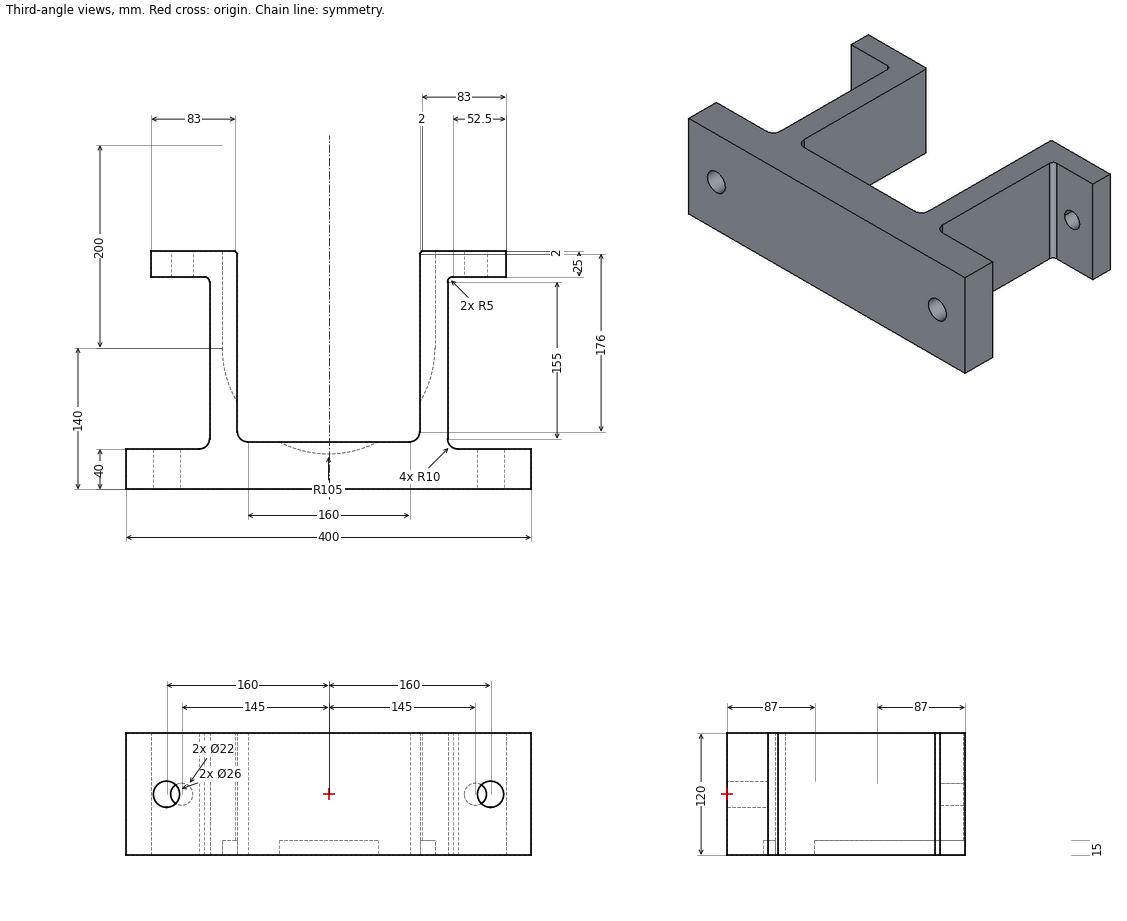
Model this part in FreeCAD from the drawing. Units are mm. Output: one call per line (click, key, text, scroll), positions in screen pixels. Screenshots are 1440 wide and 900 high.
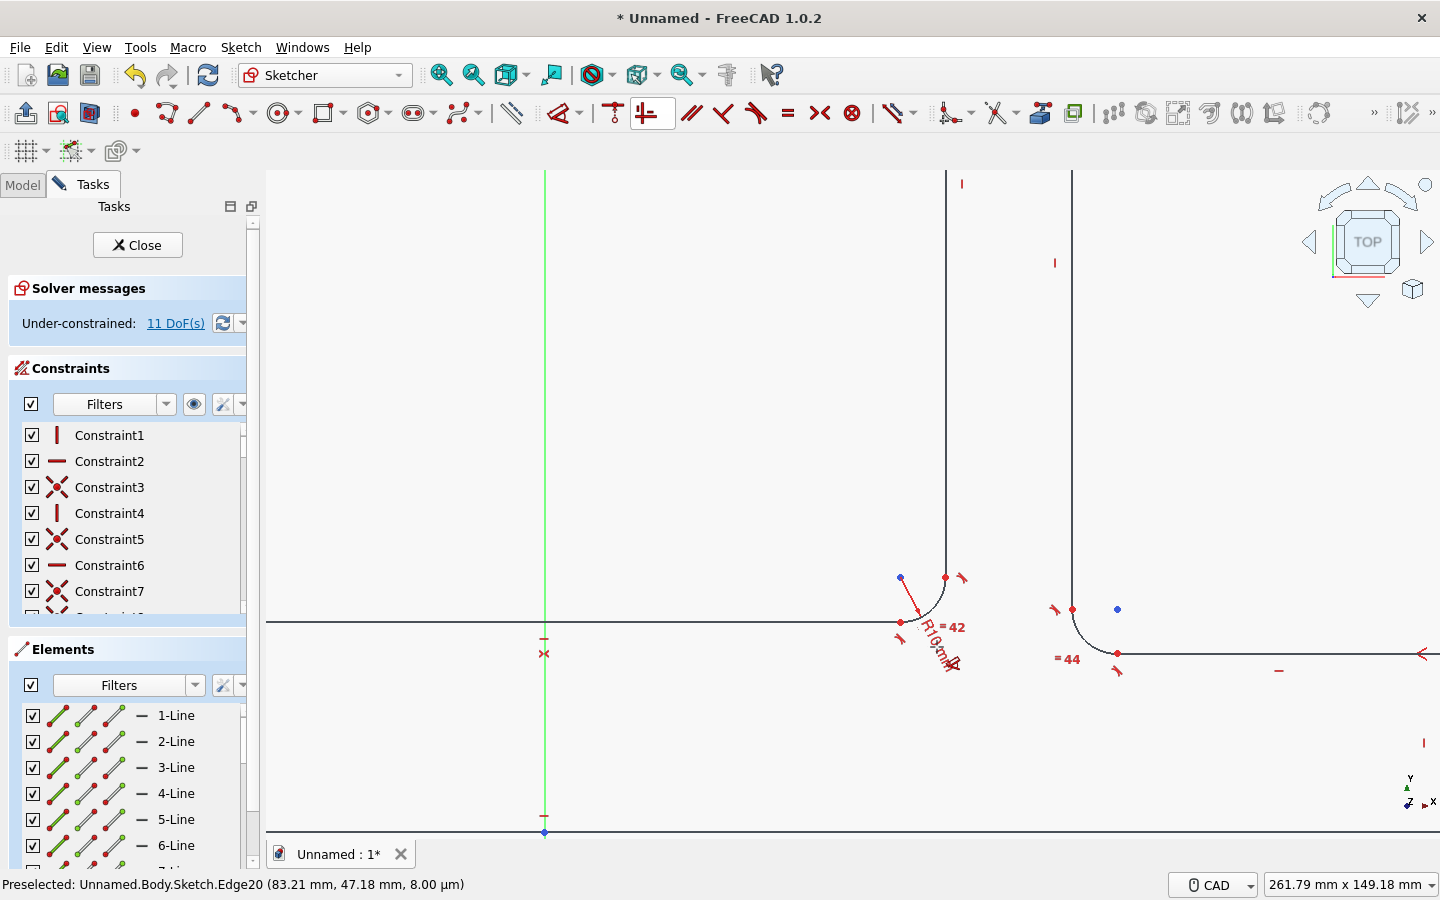
scroll(924, 621, down, 5)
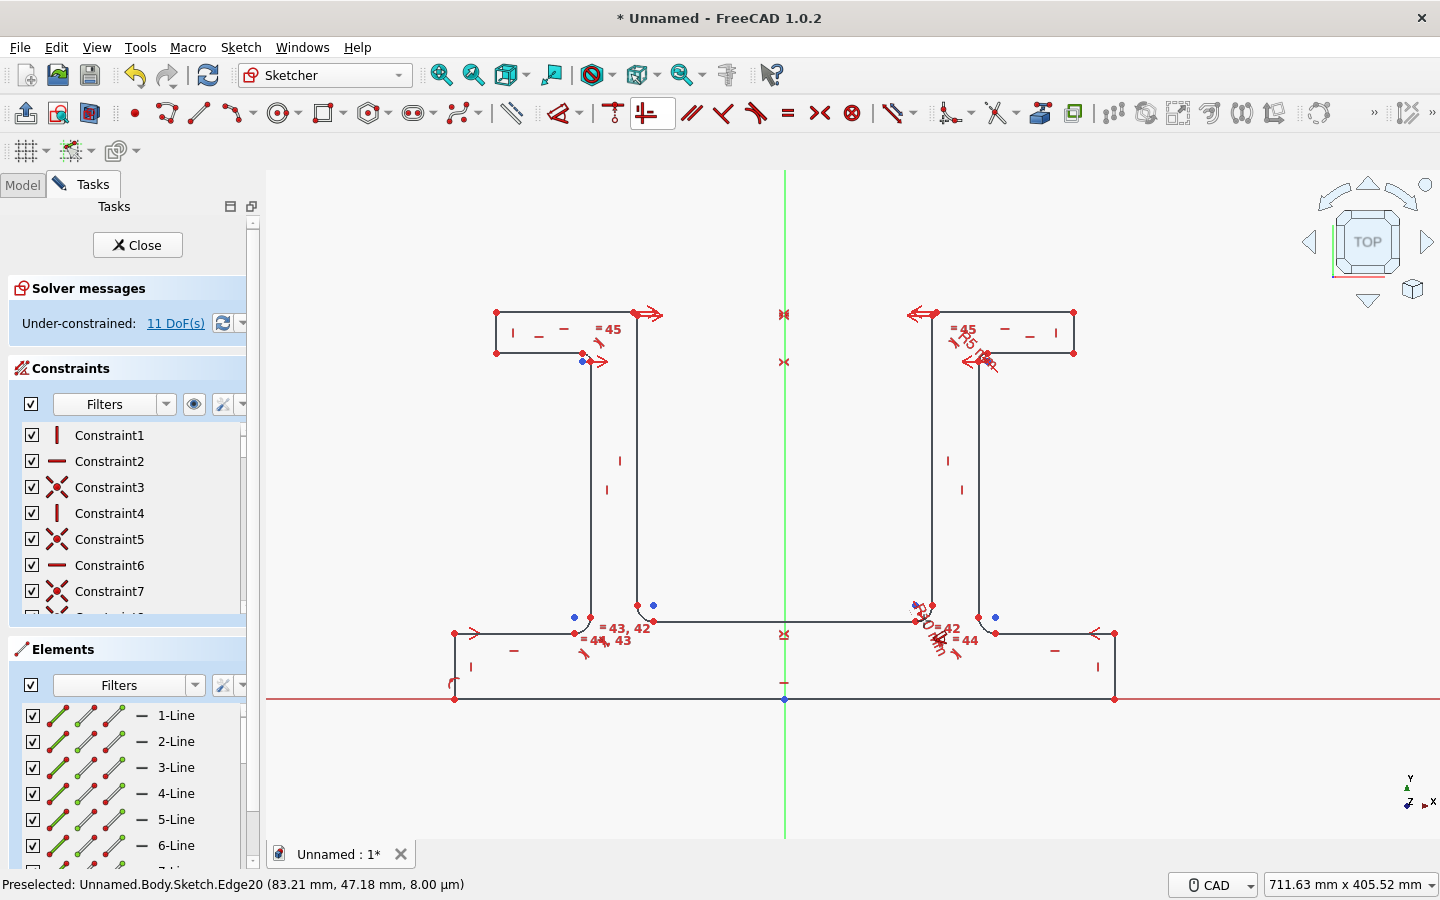
click(1074, 341)
click(1108, 333)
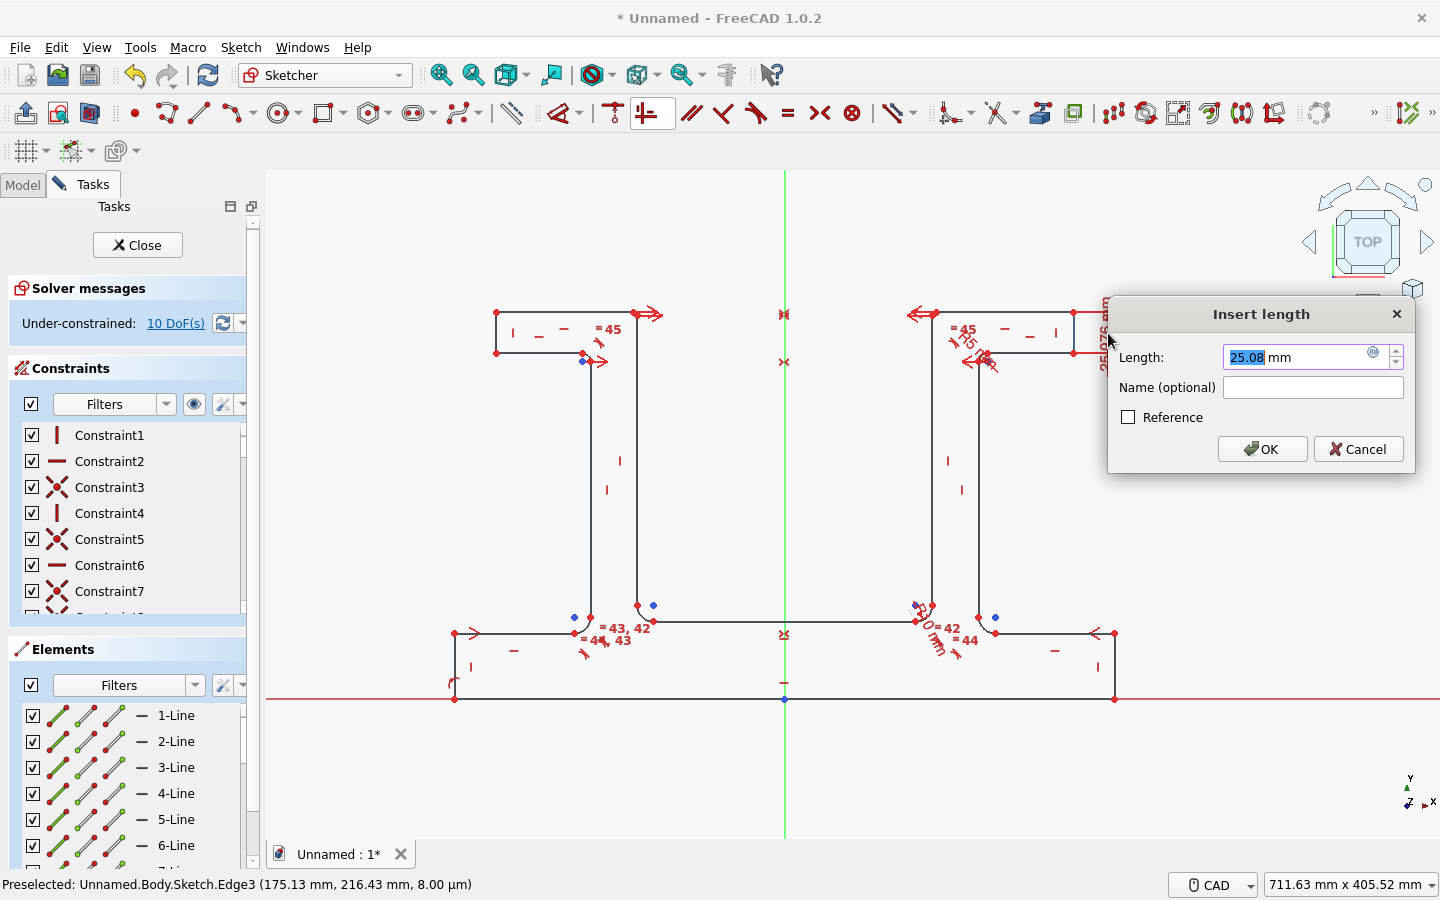
text(25)
key(Return)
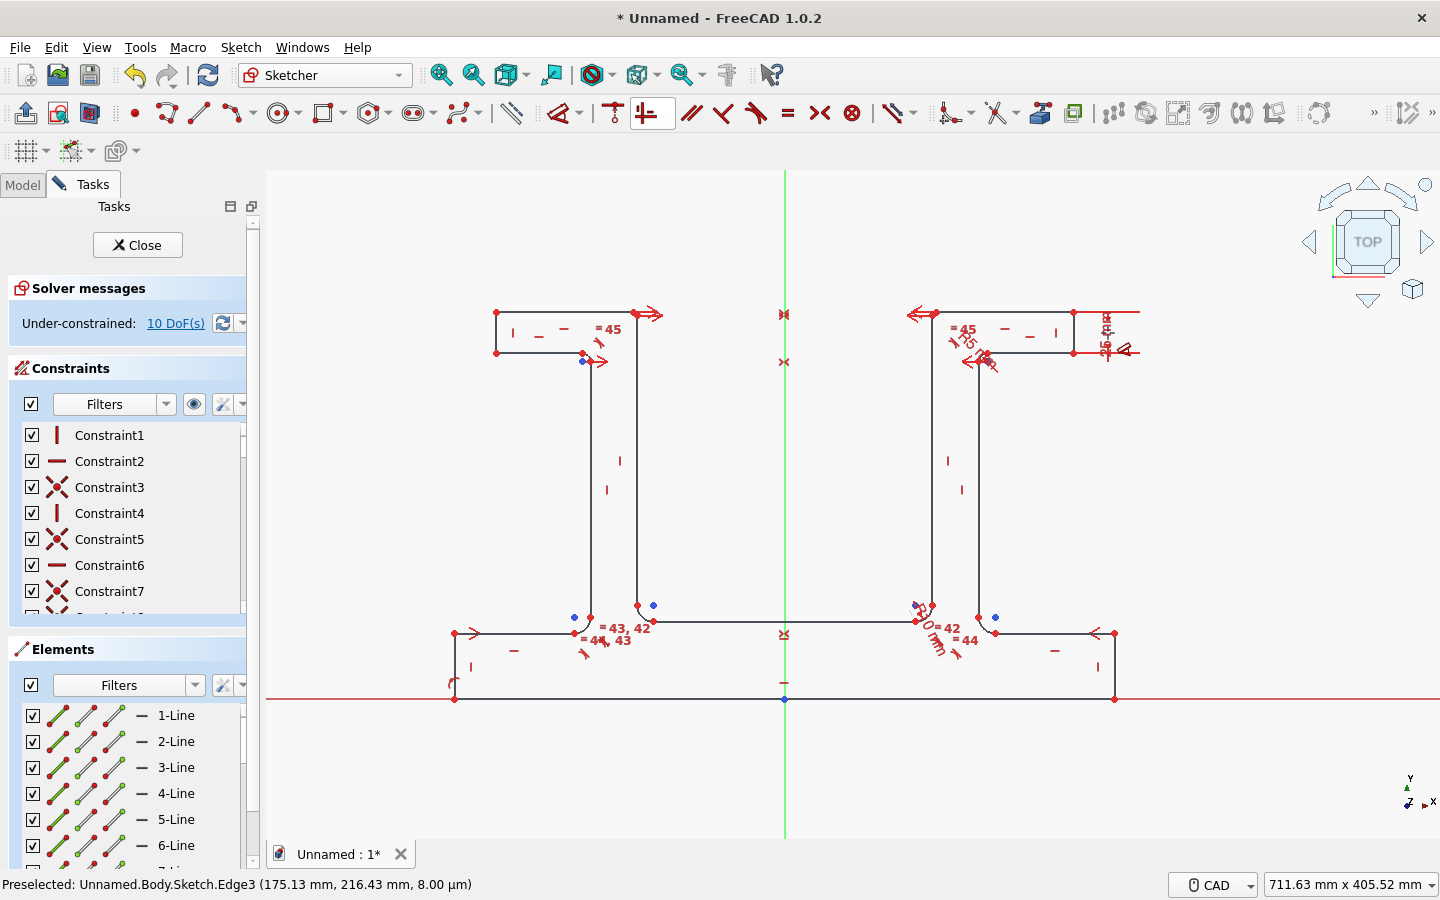
click(1032, 312)
click(1005, 278)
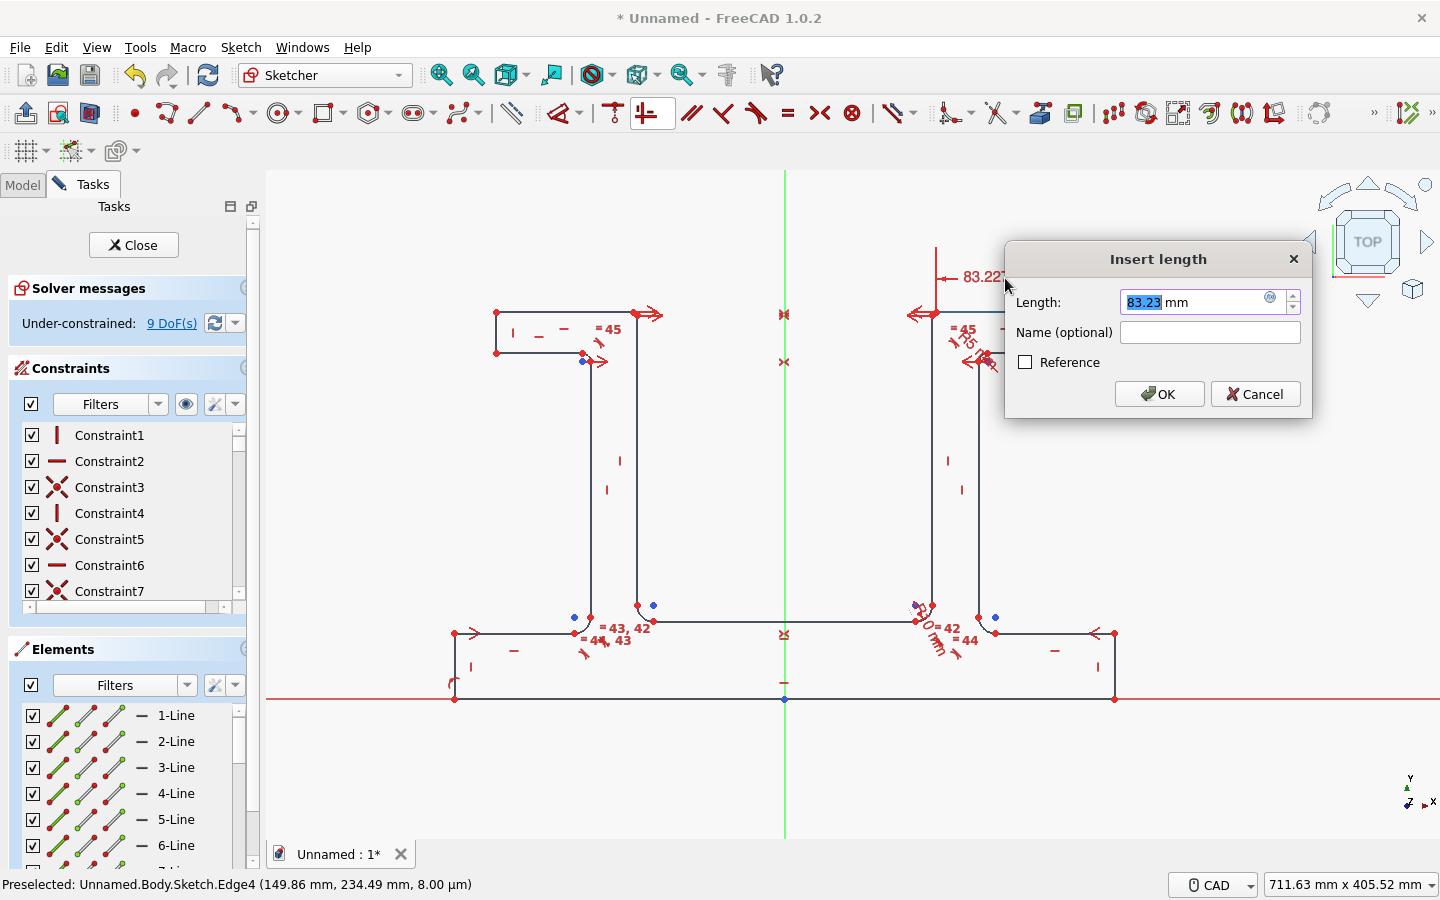
text(83)
key(Return)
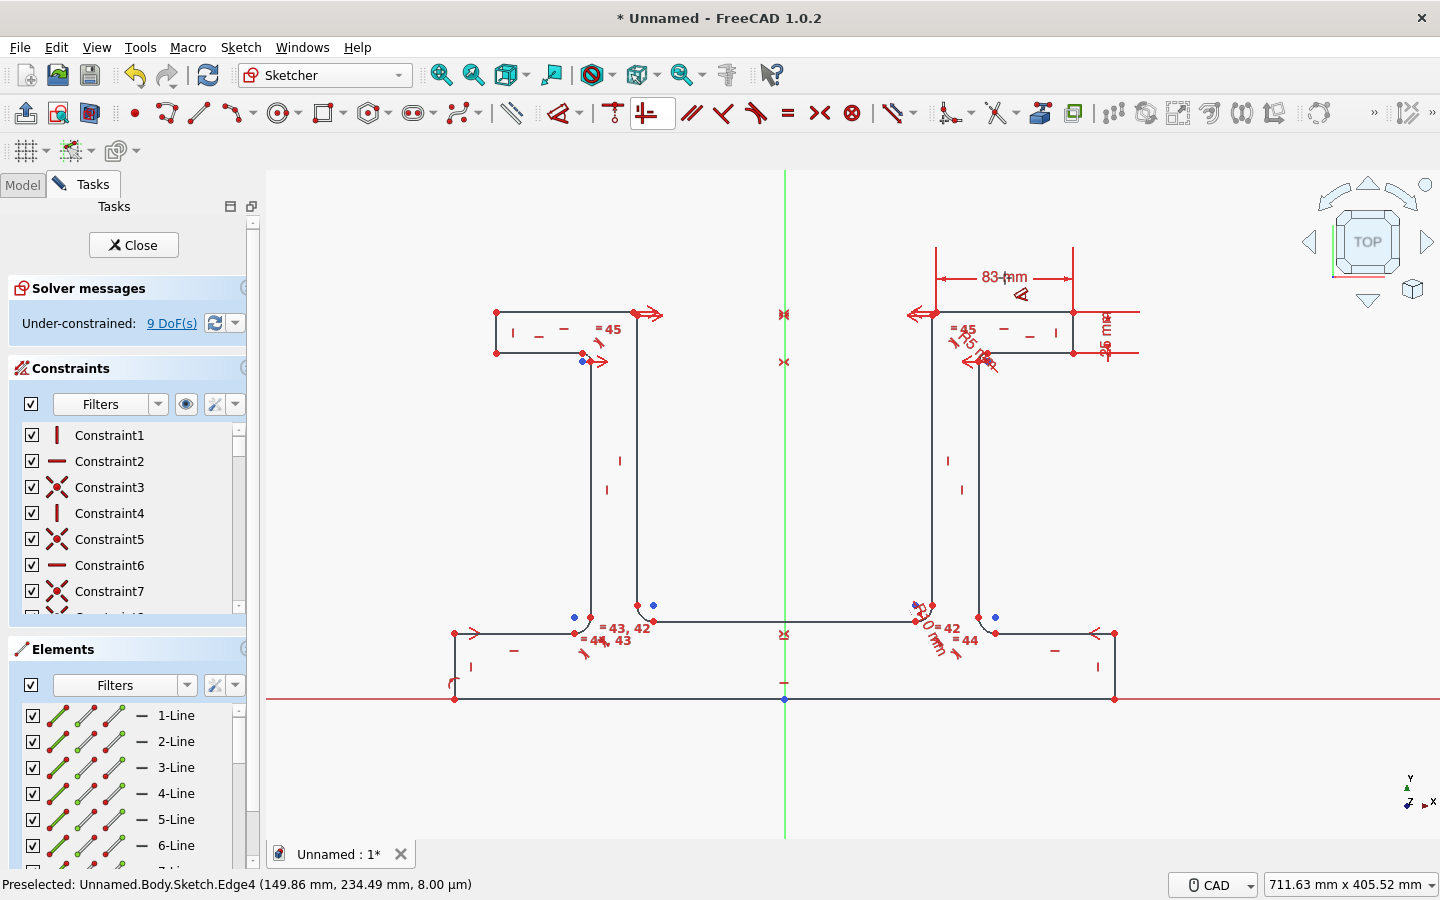
click(592, 312)
click(565, 278)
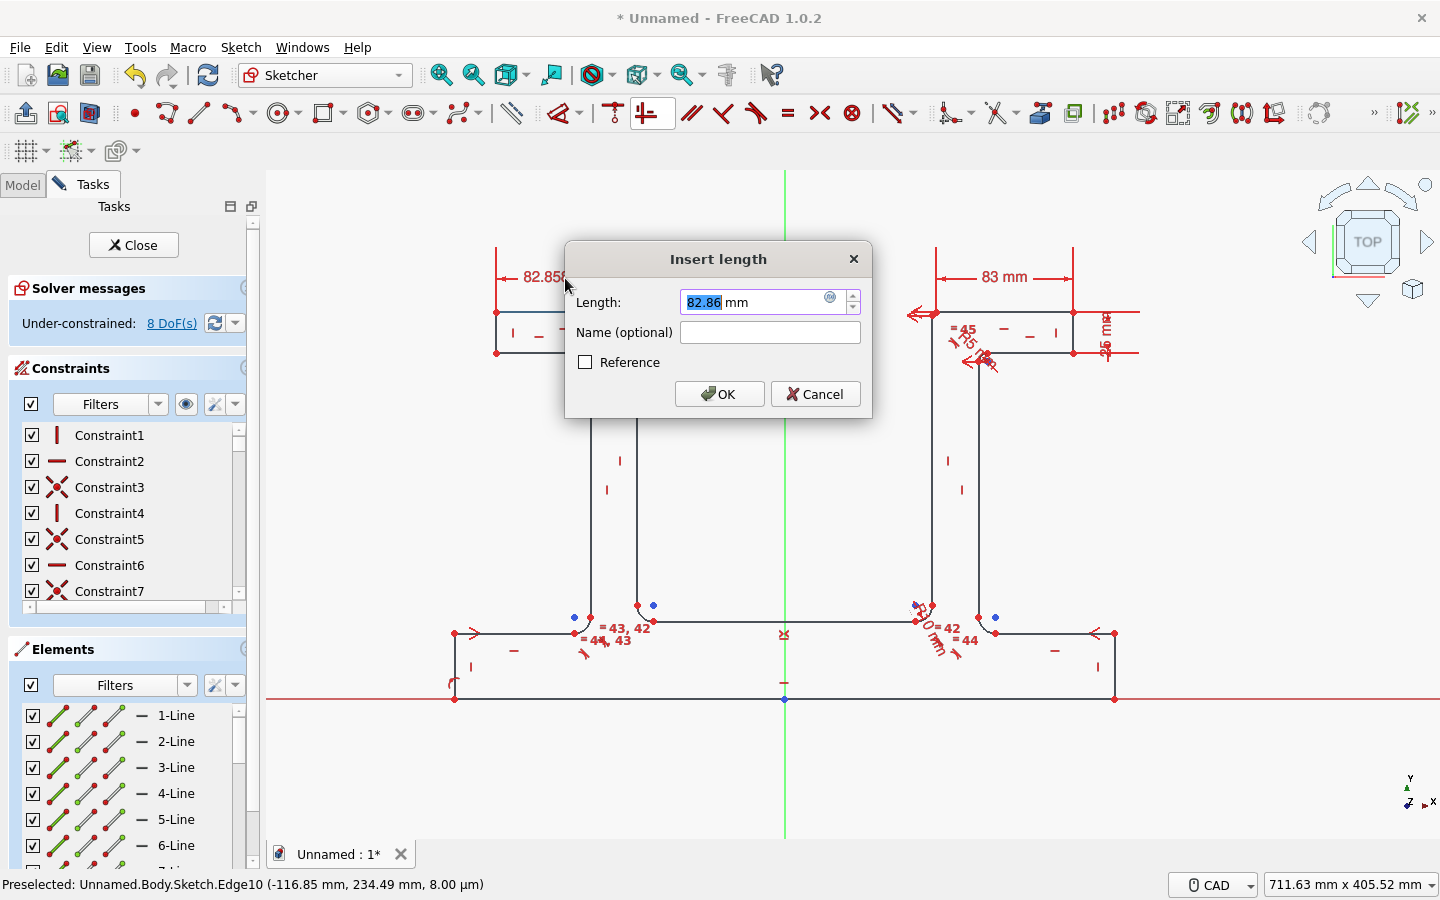
text(83)
key(Return)